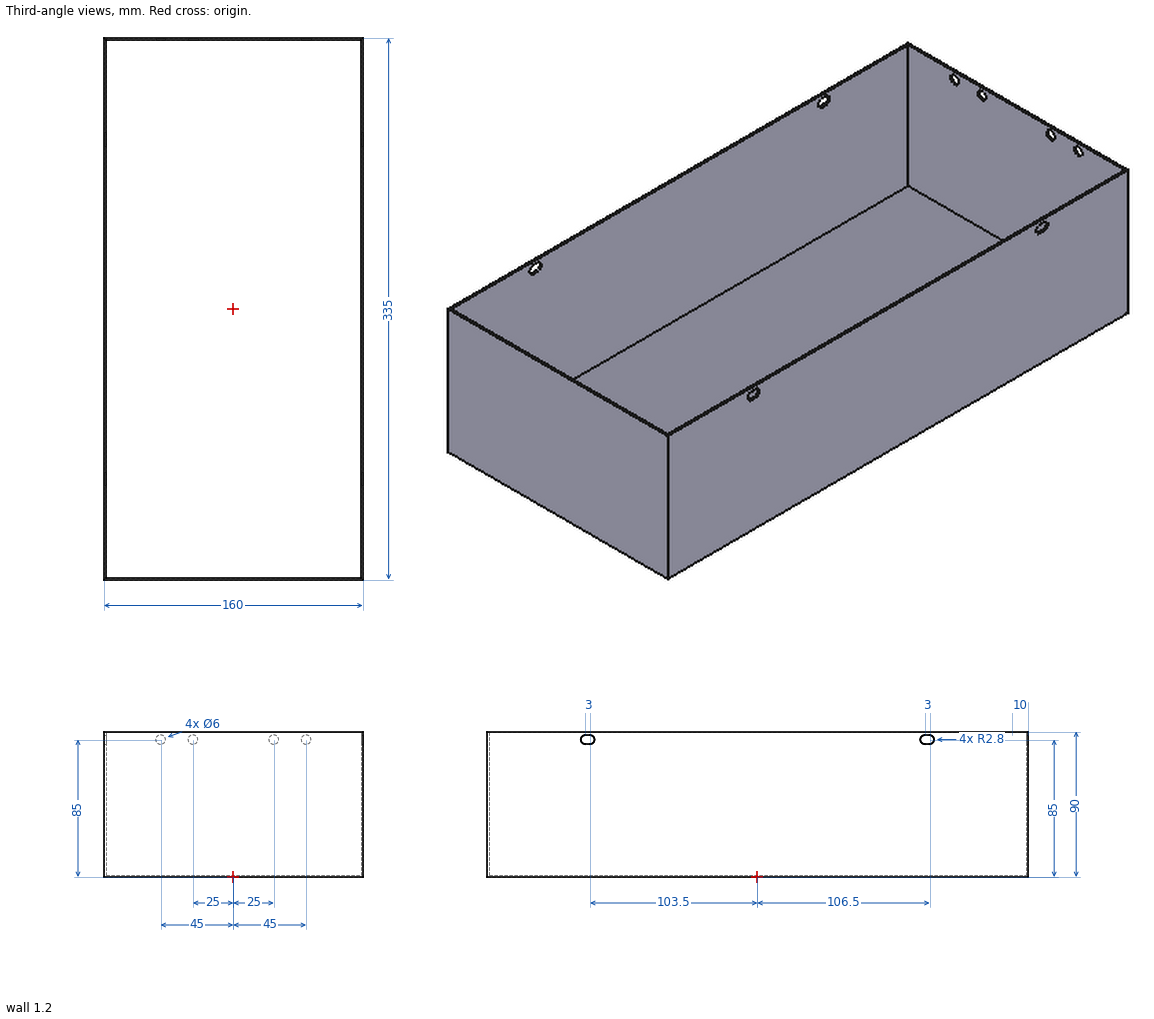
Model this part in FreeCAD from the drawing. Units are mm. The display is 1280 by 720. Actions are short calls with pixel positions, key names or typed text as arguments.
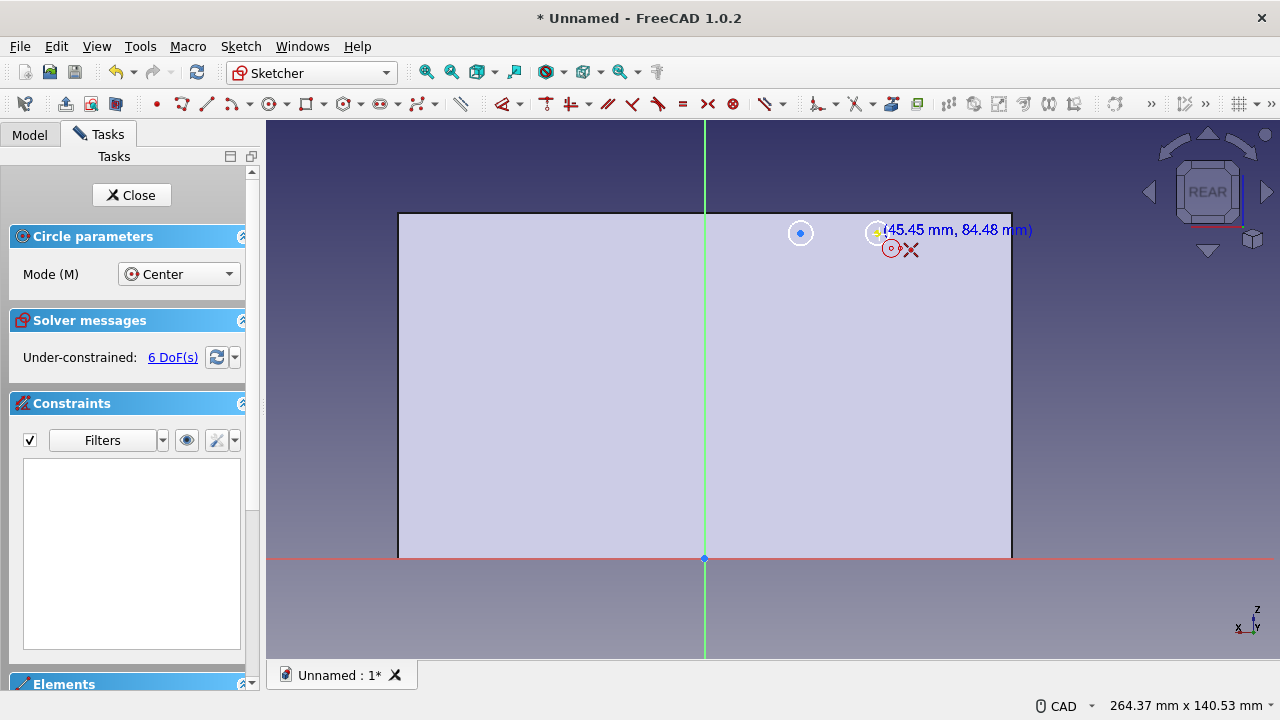
scroll(609, 233, up, 4)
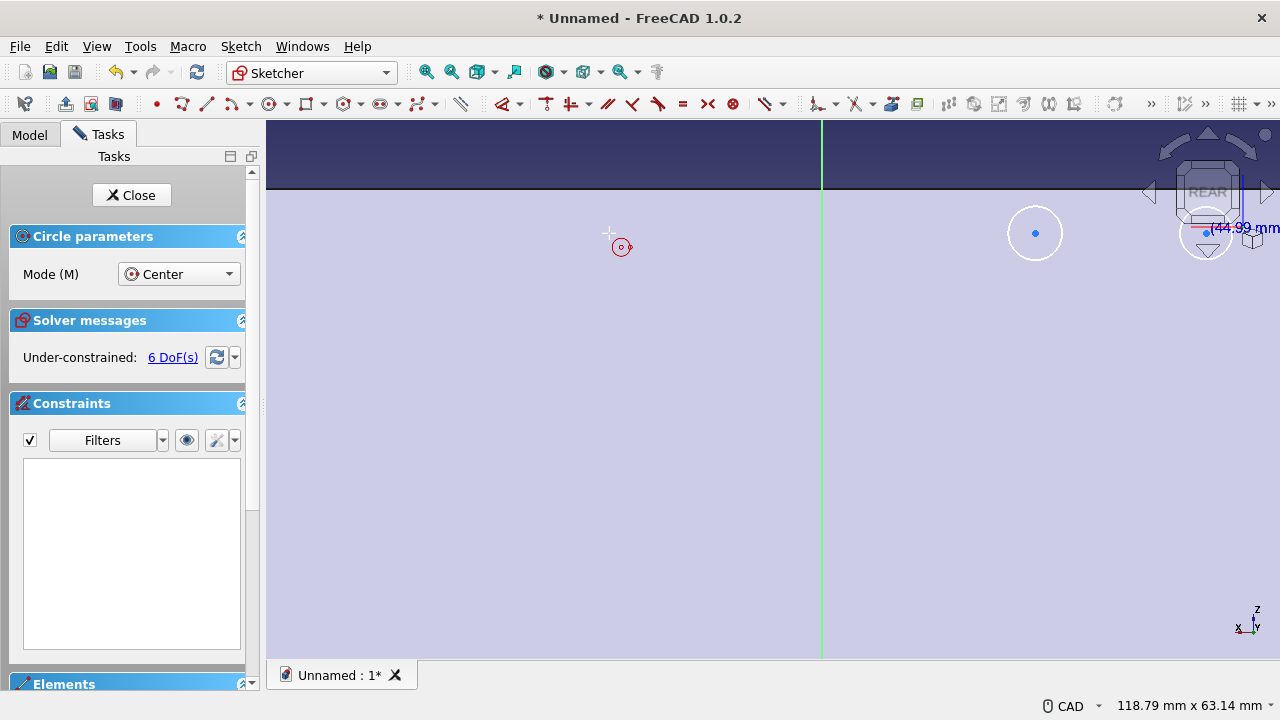
click(609, 232)
click(627, 214)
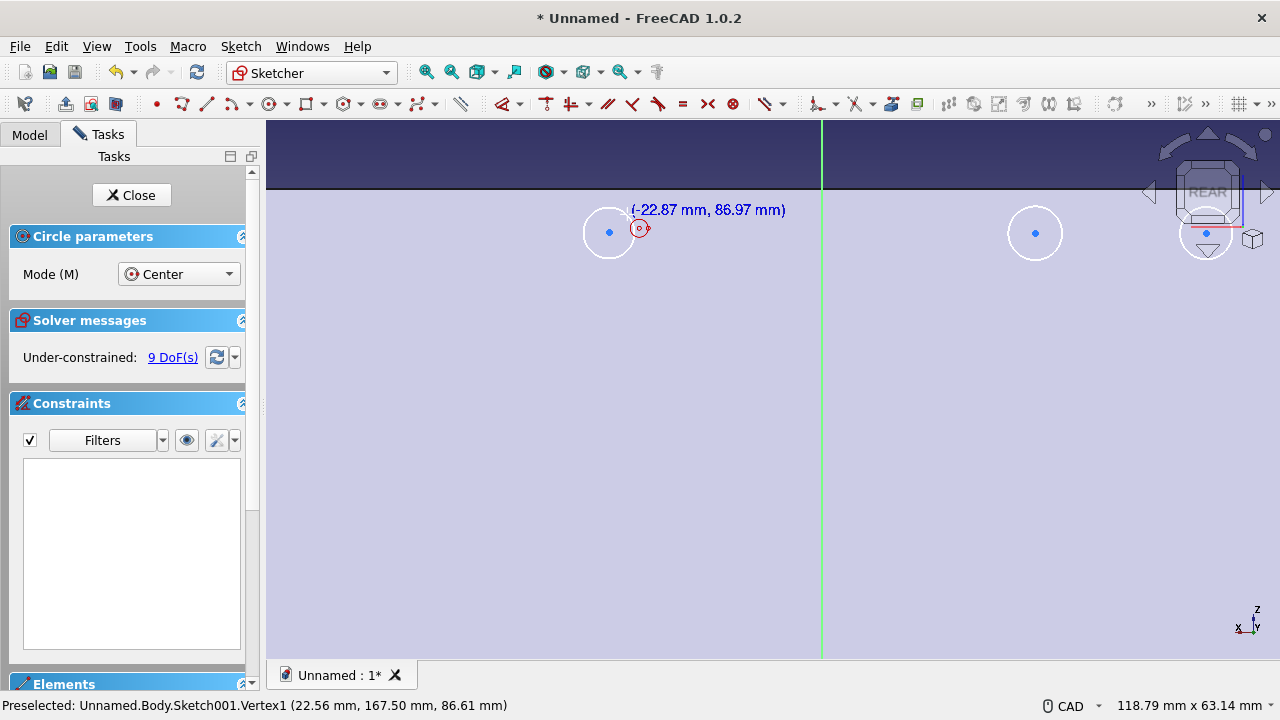
click(438, 232)
click(456, 214)
key(Escape)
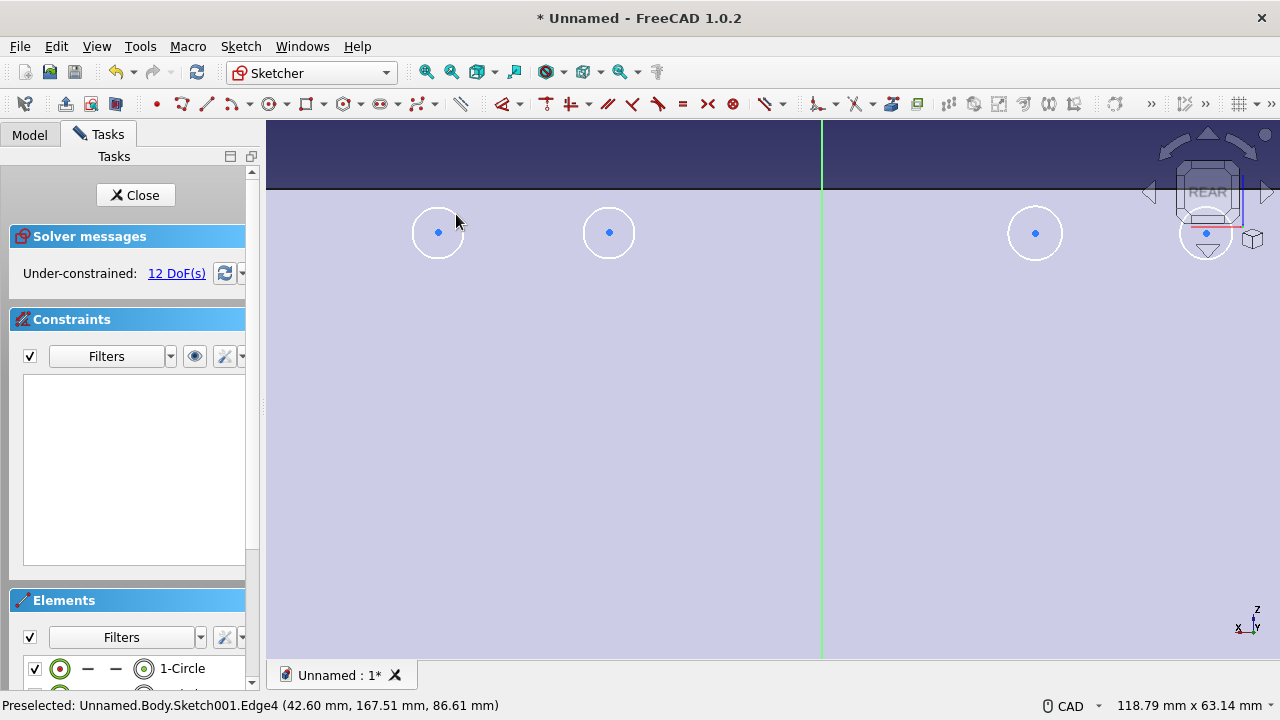
scroll(608, 233, down, 4)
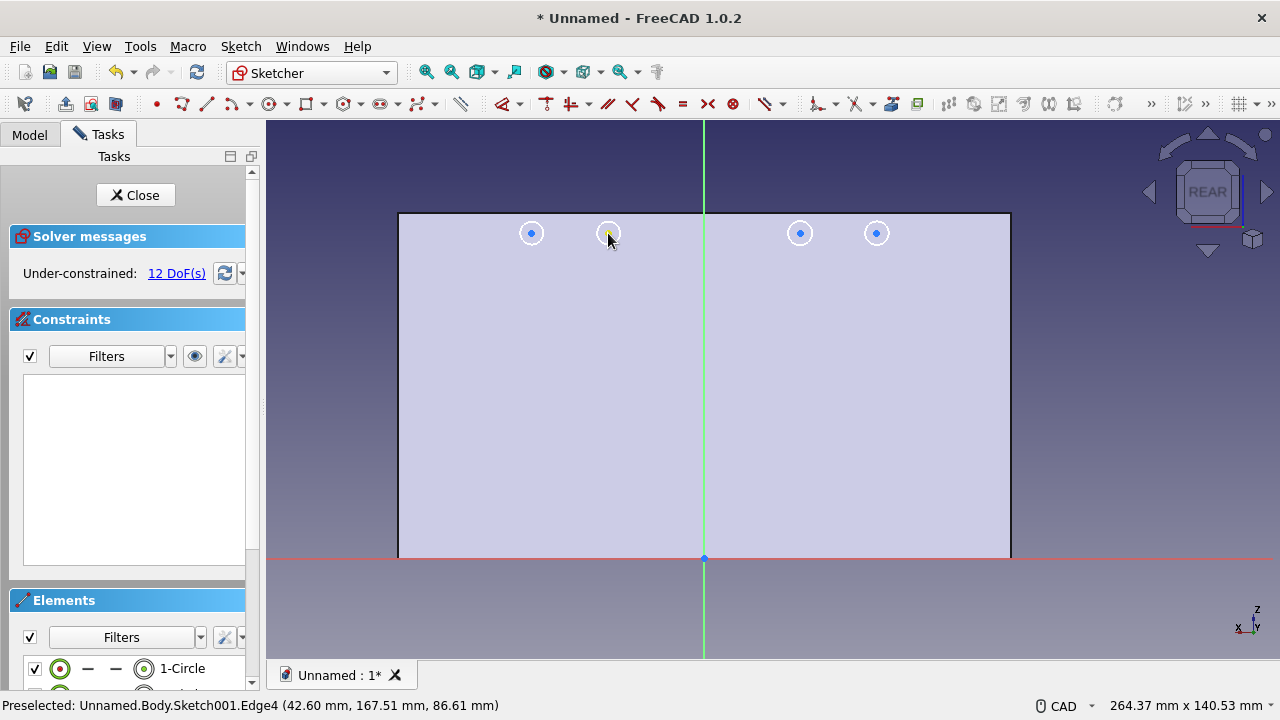
click(885, 225)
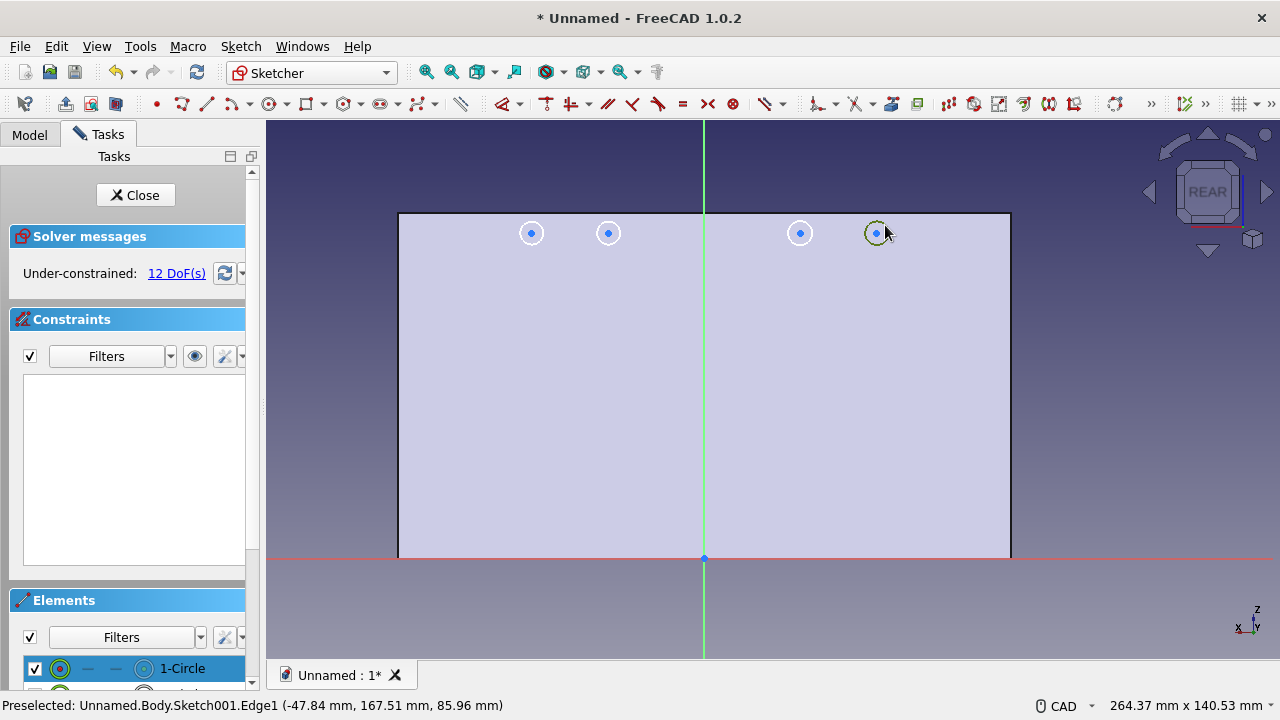
click(809, 225)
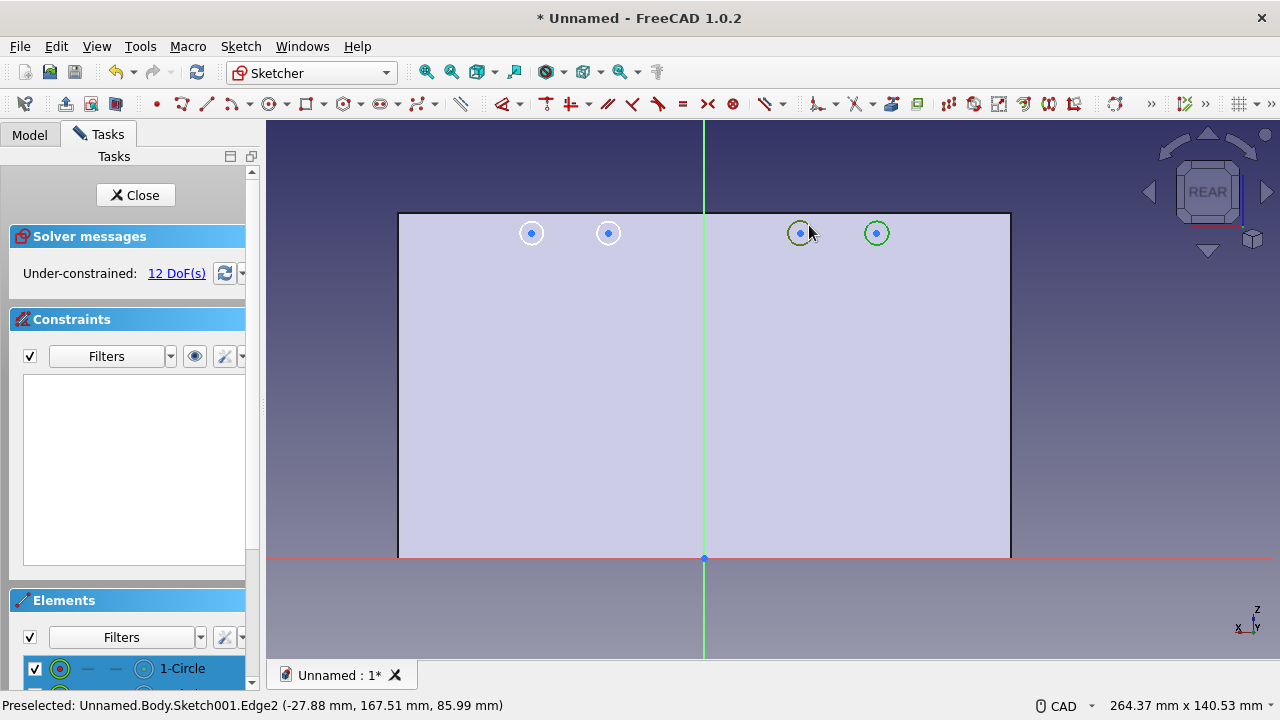
click(617, 225)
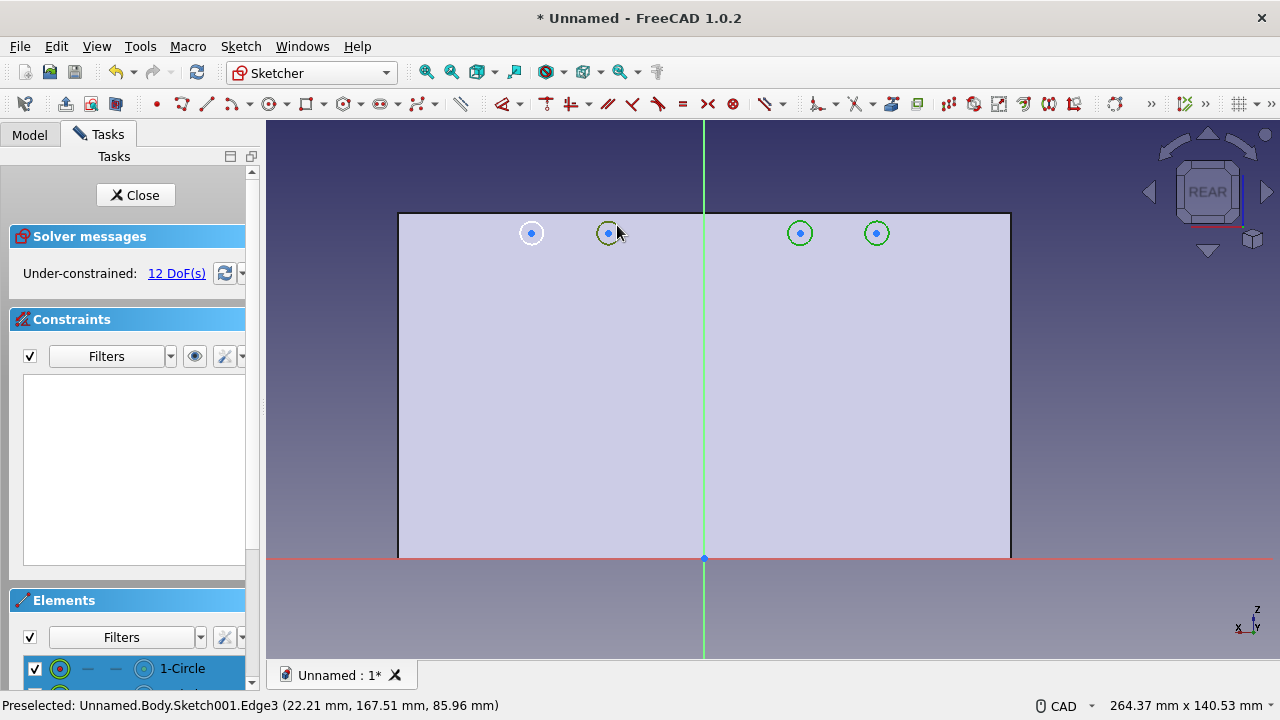
click(540, 225)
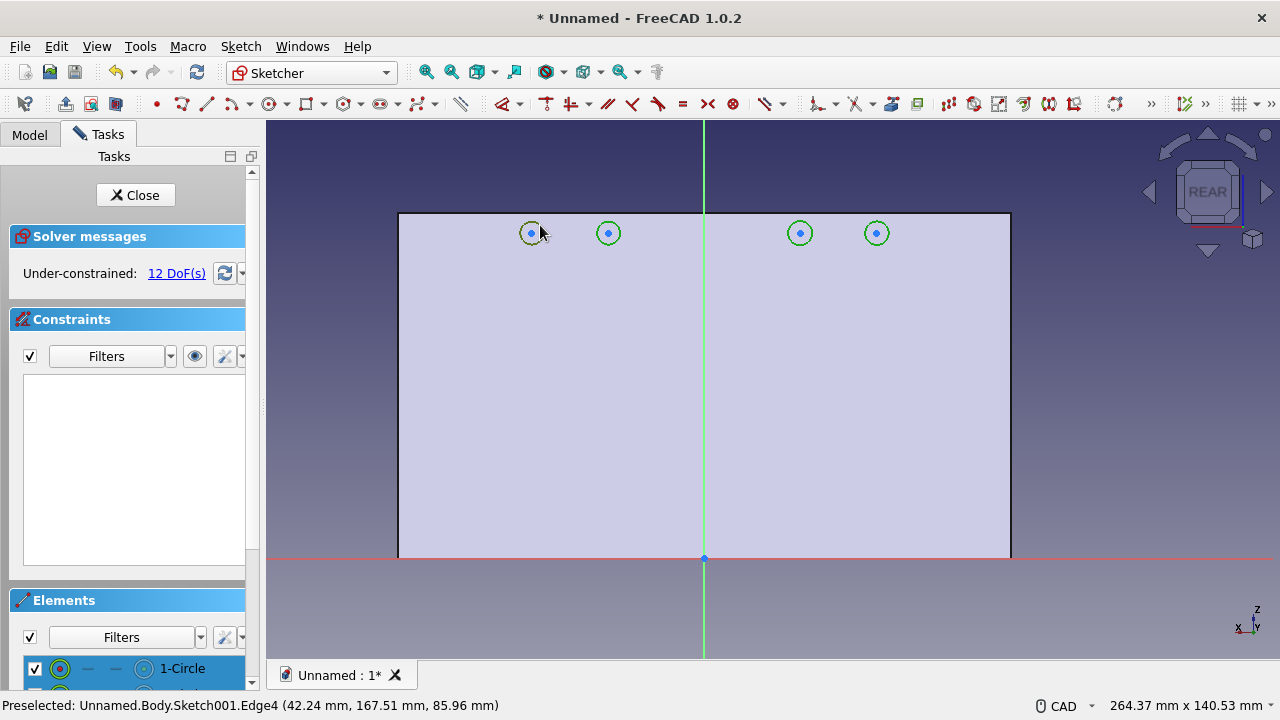
click(683, 104)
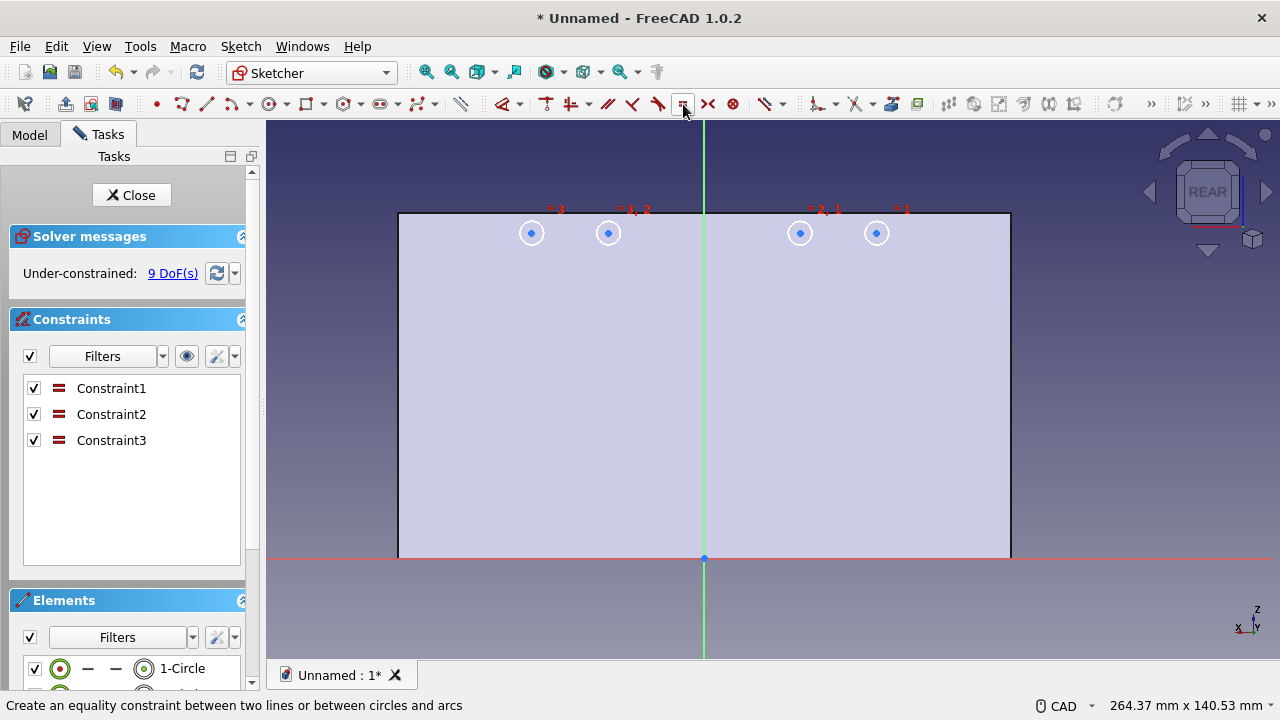
click(877, 233)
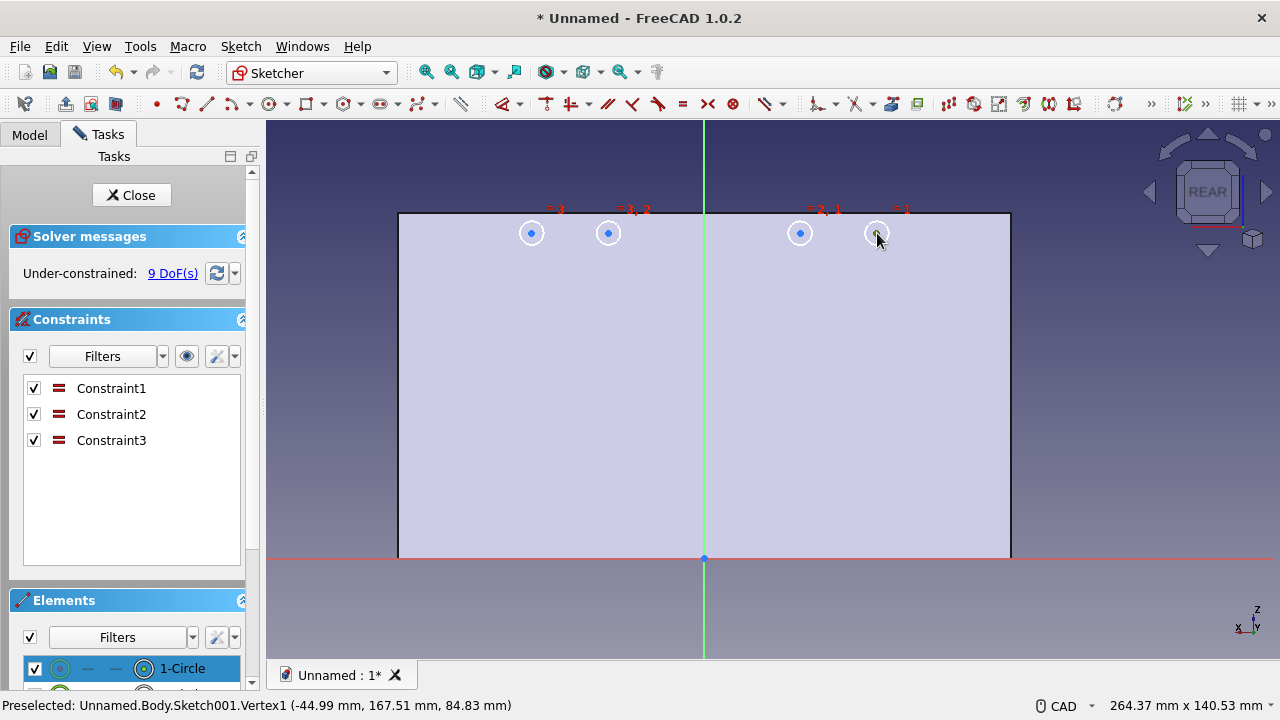
click(800, 233)